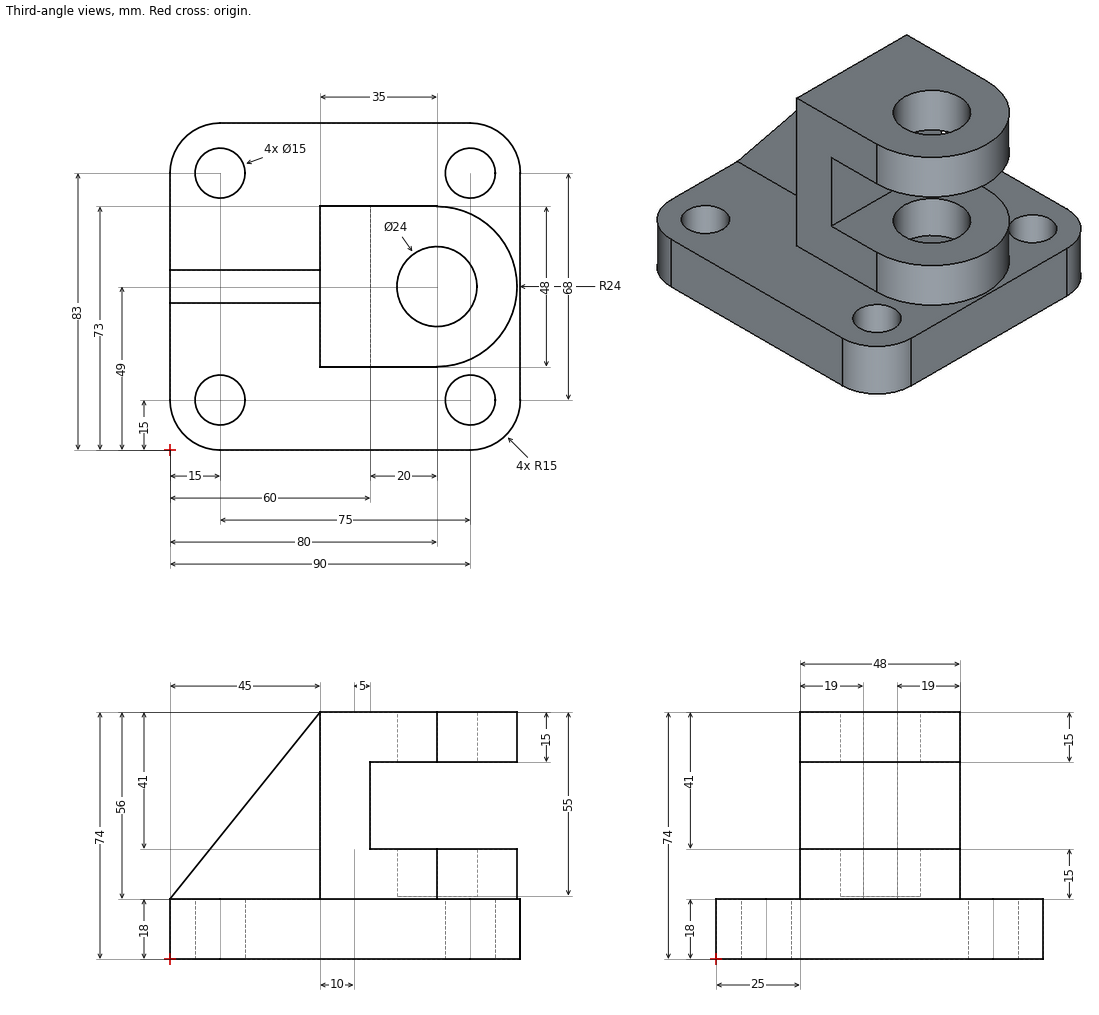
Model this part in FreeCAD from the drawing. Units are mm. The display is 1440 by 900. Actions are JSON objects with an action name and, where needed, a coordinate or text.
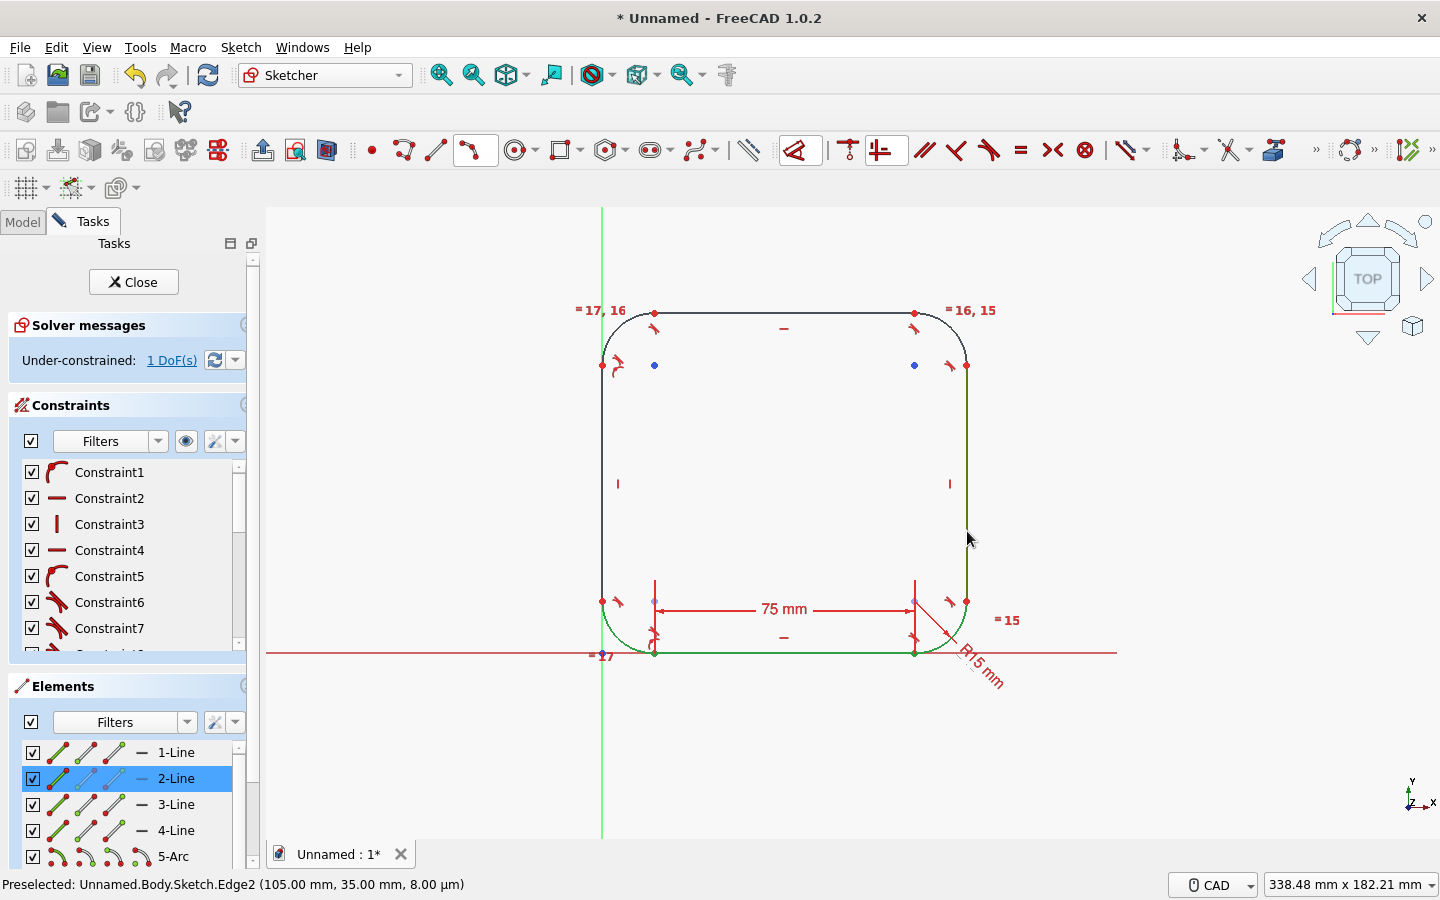
{"action": "key", "text": "i"}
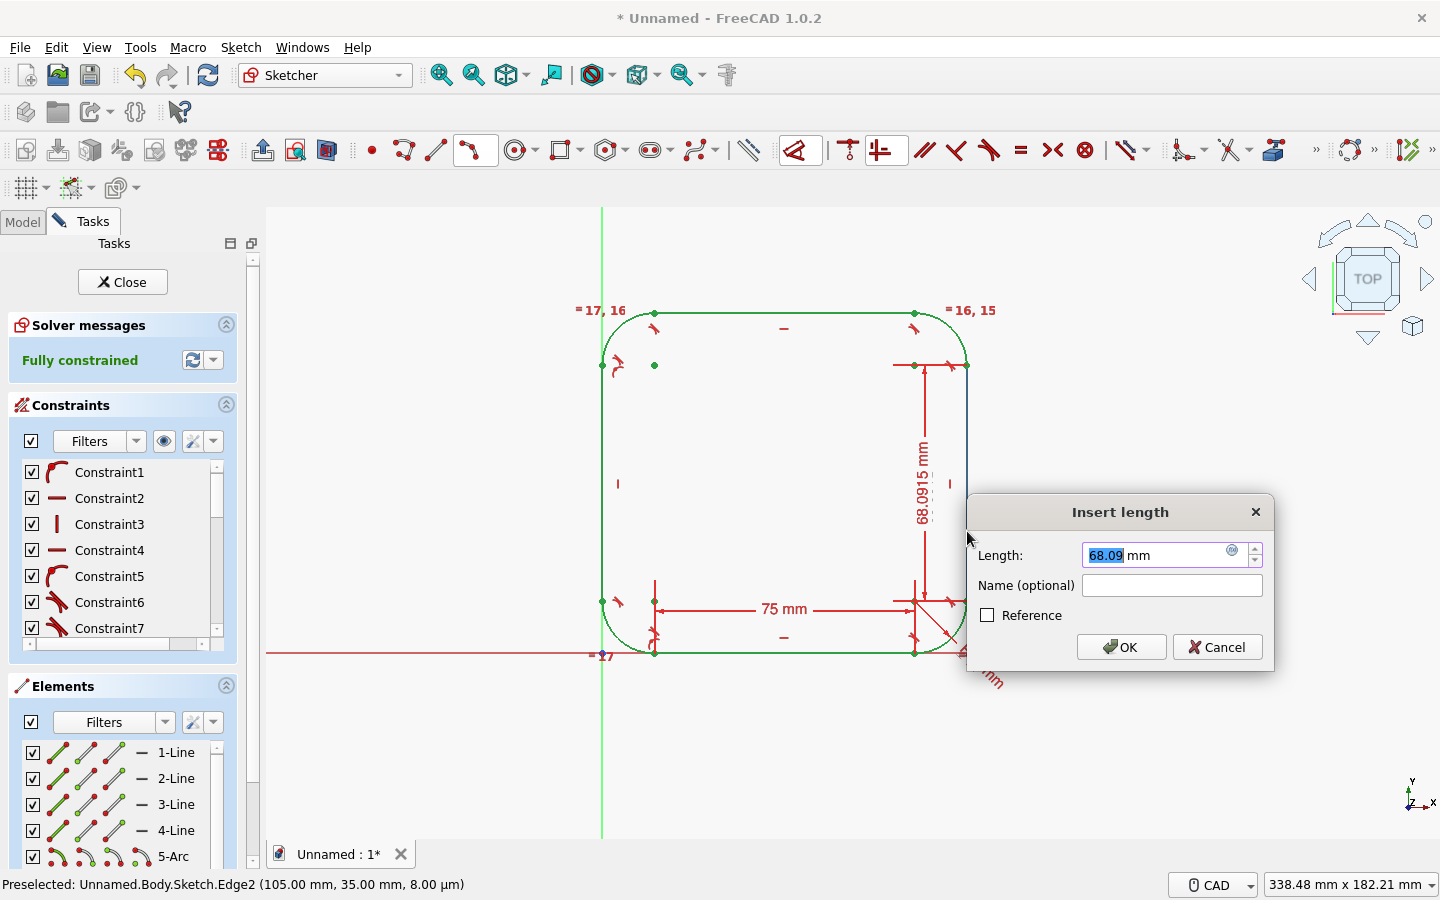
{"action": "type", "text": "68"}
{"action": "key", "text": "Return"}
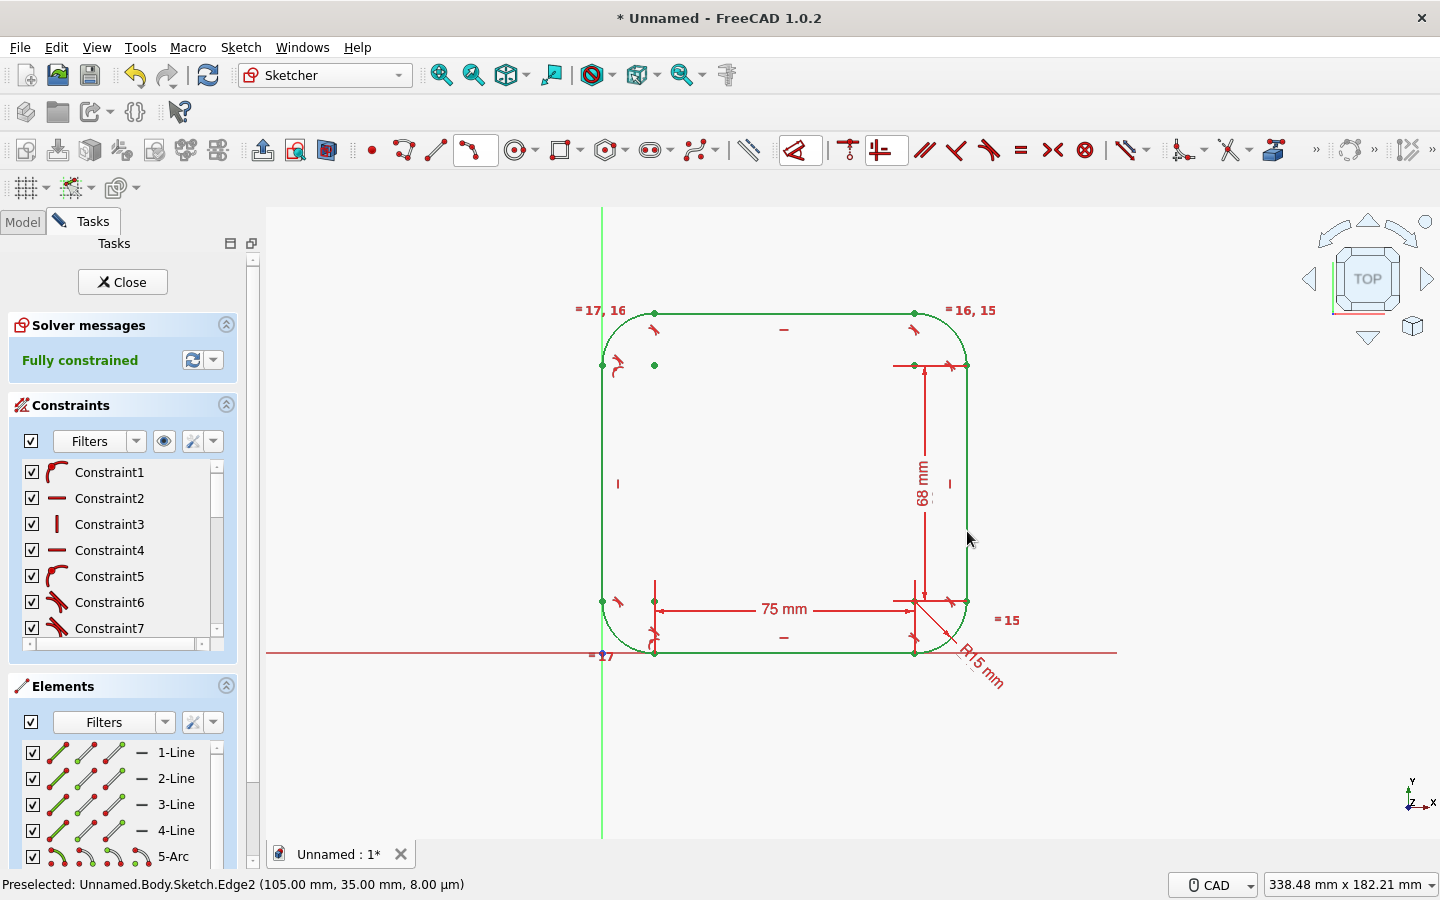
{"action": "left_click", "coordinate": [123, 282]}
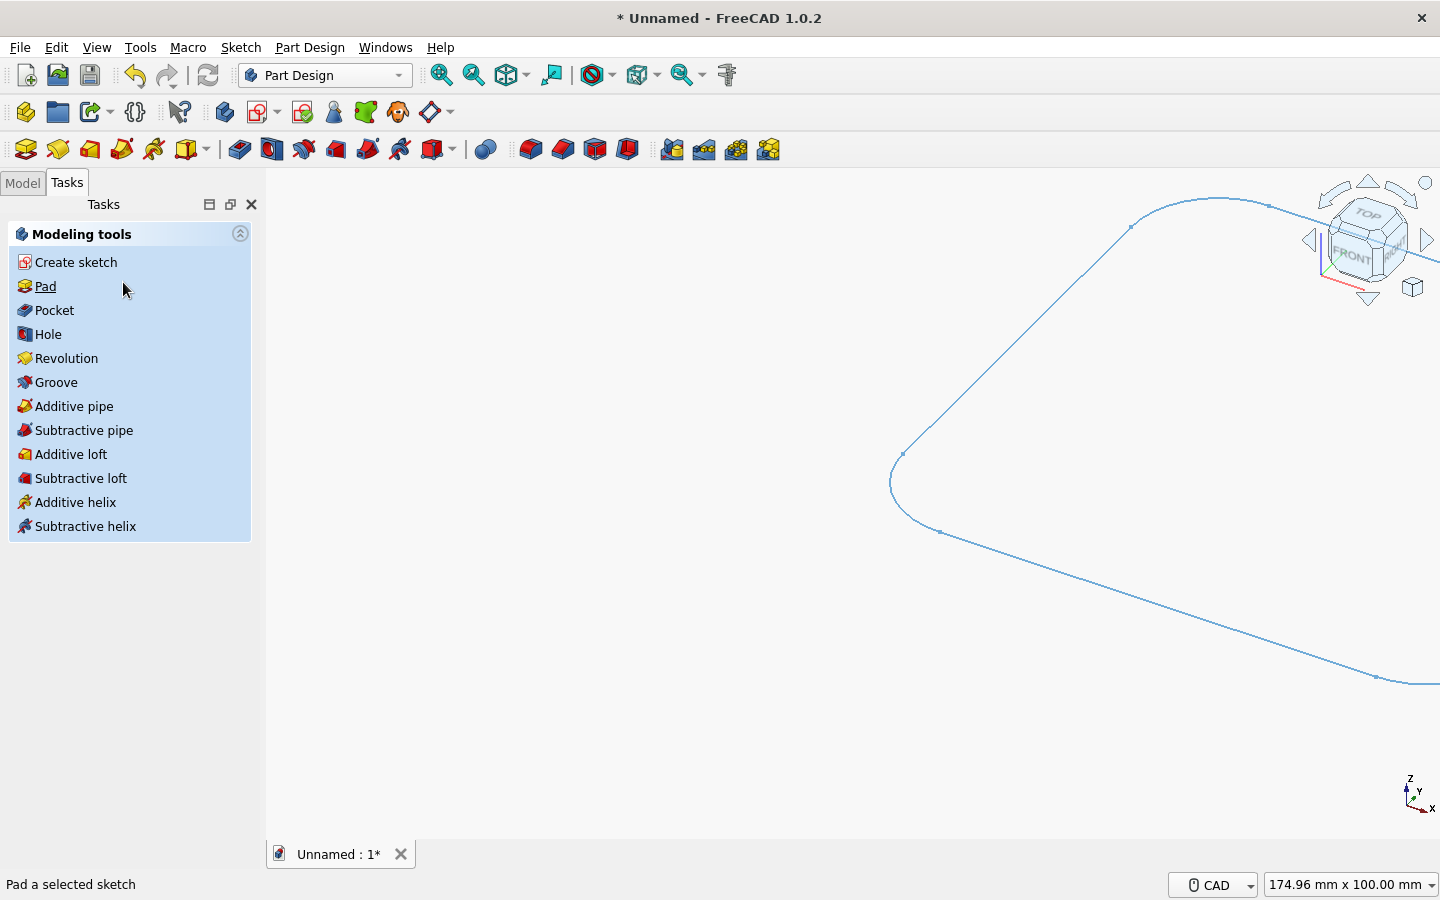
{"action": "left_click", "coordinate": [26, 150]}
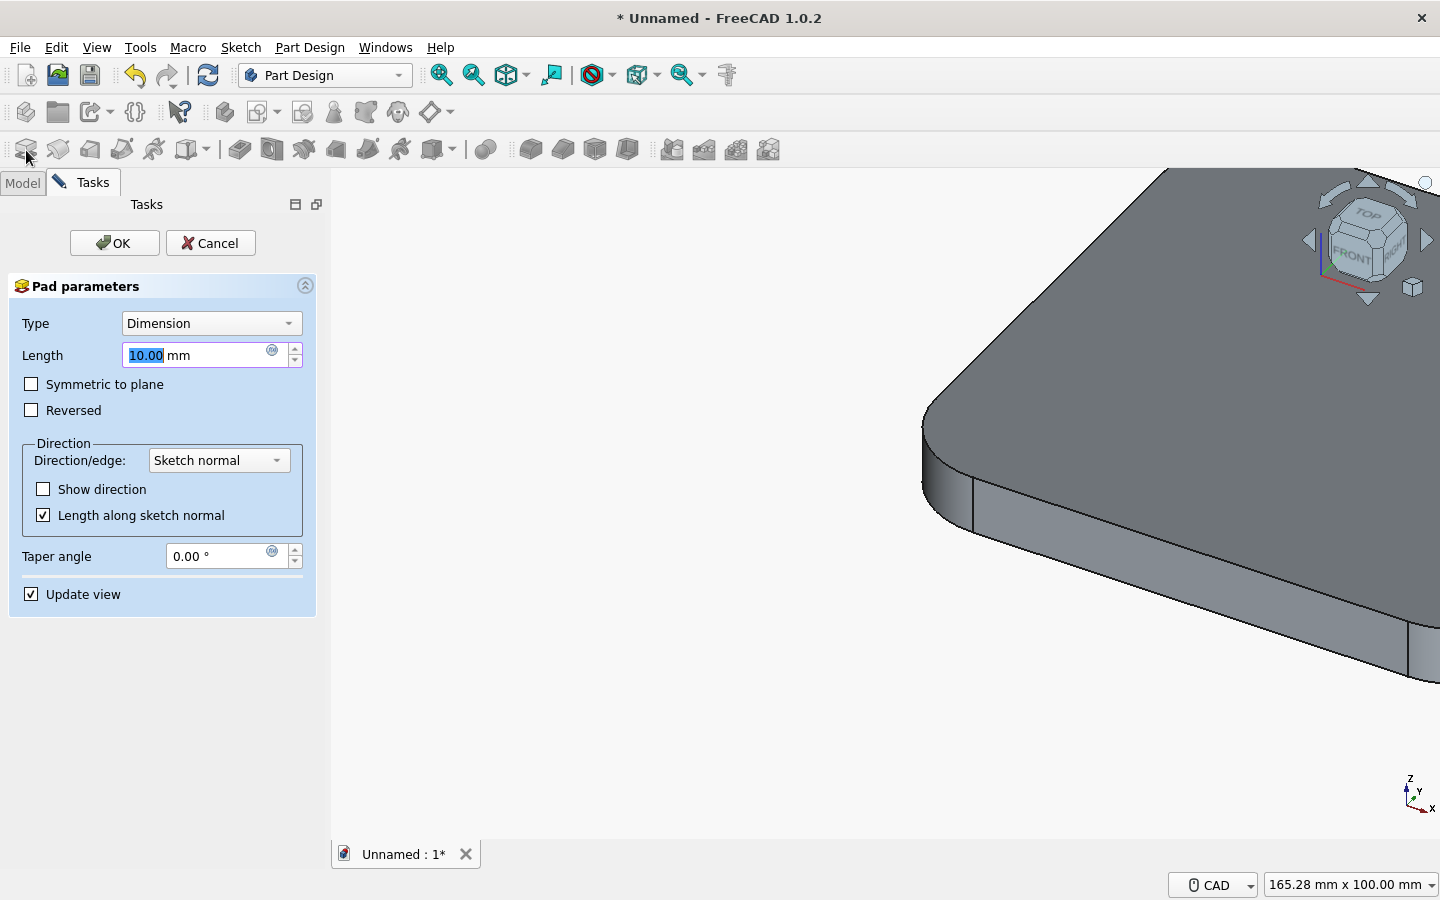
{"action": "type", "text": "18"}
{"action": "key", "text": "Tab"}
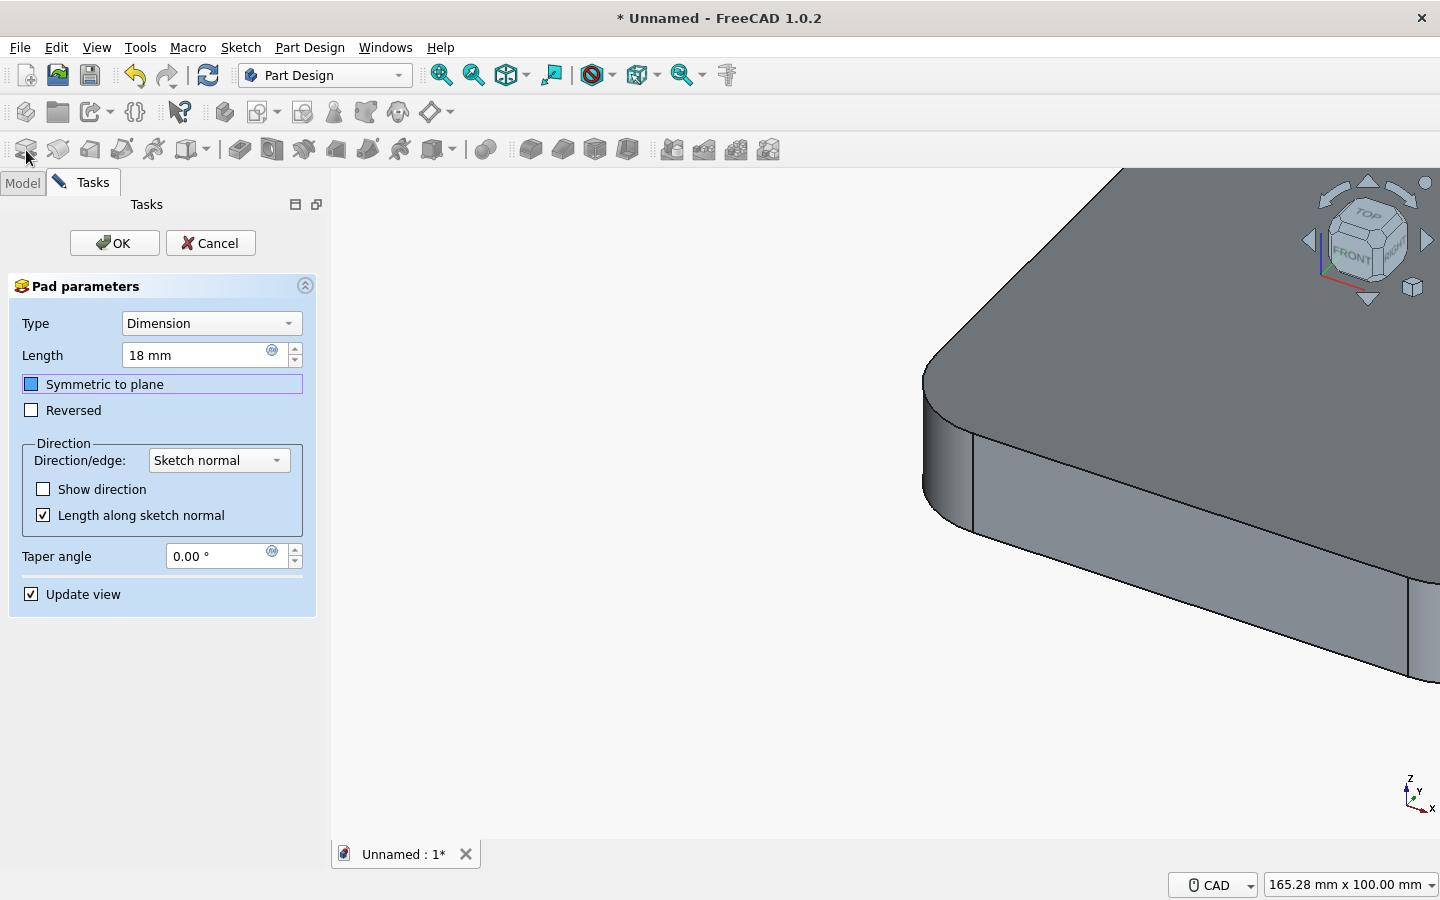
{"action": "left_click", "coordinate": [115, 243]}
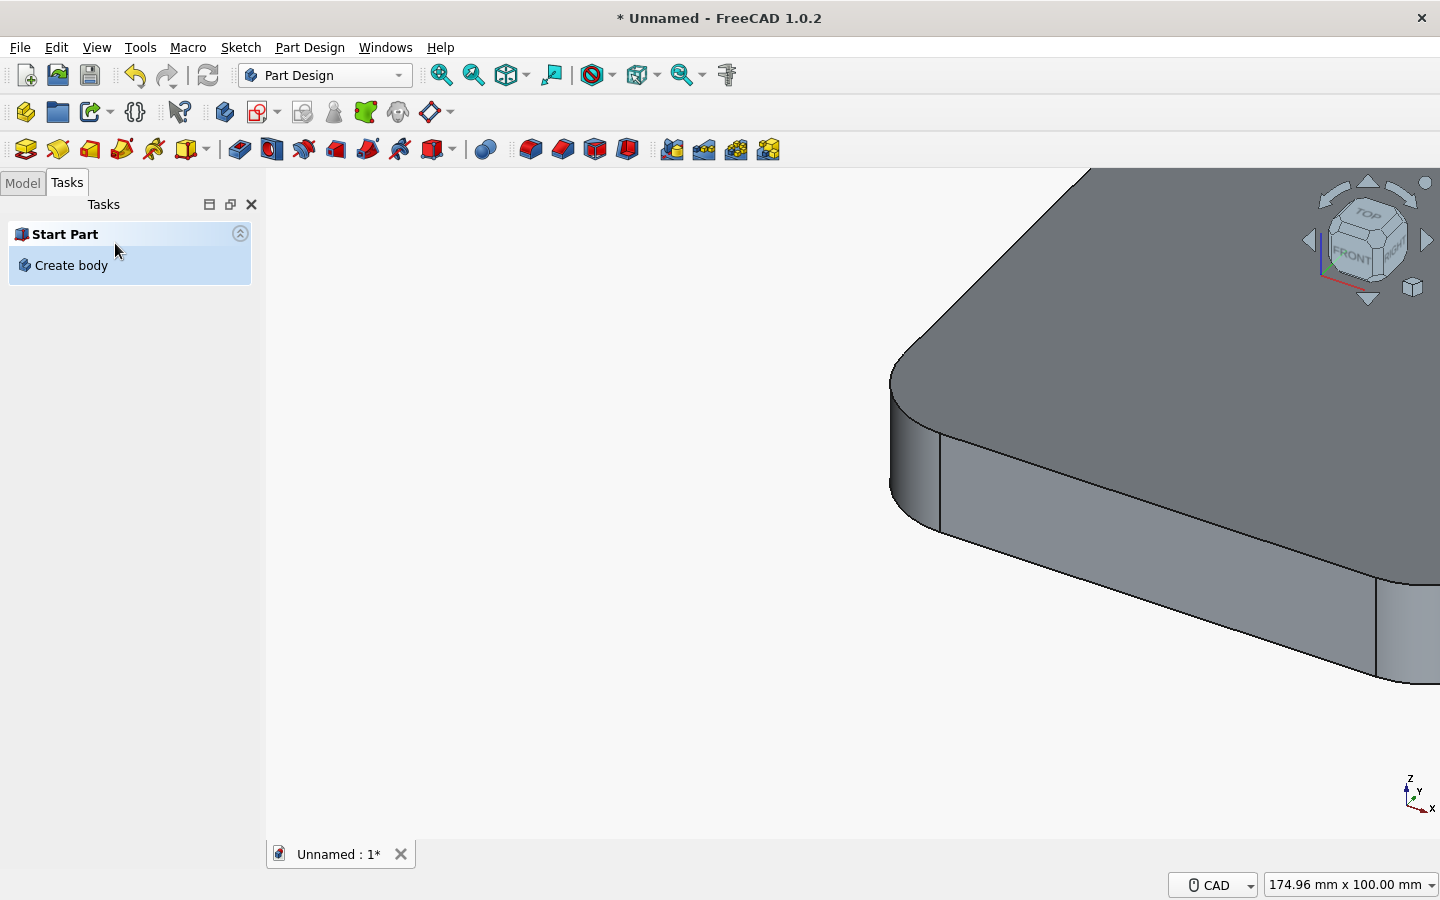
{"action": "left_click", "coordinate": [442, 76]}